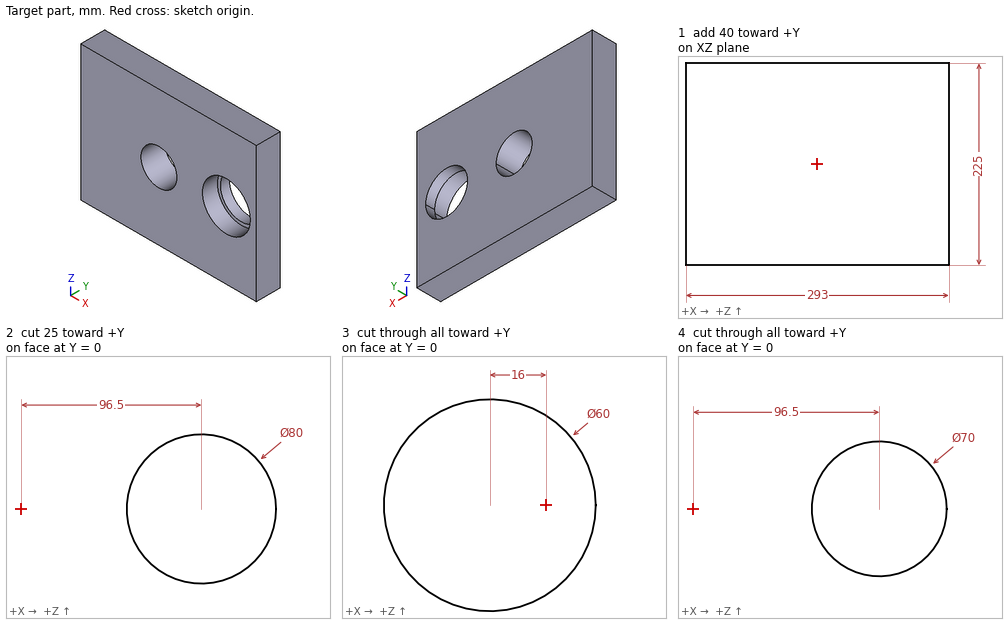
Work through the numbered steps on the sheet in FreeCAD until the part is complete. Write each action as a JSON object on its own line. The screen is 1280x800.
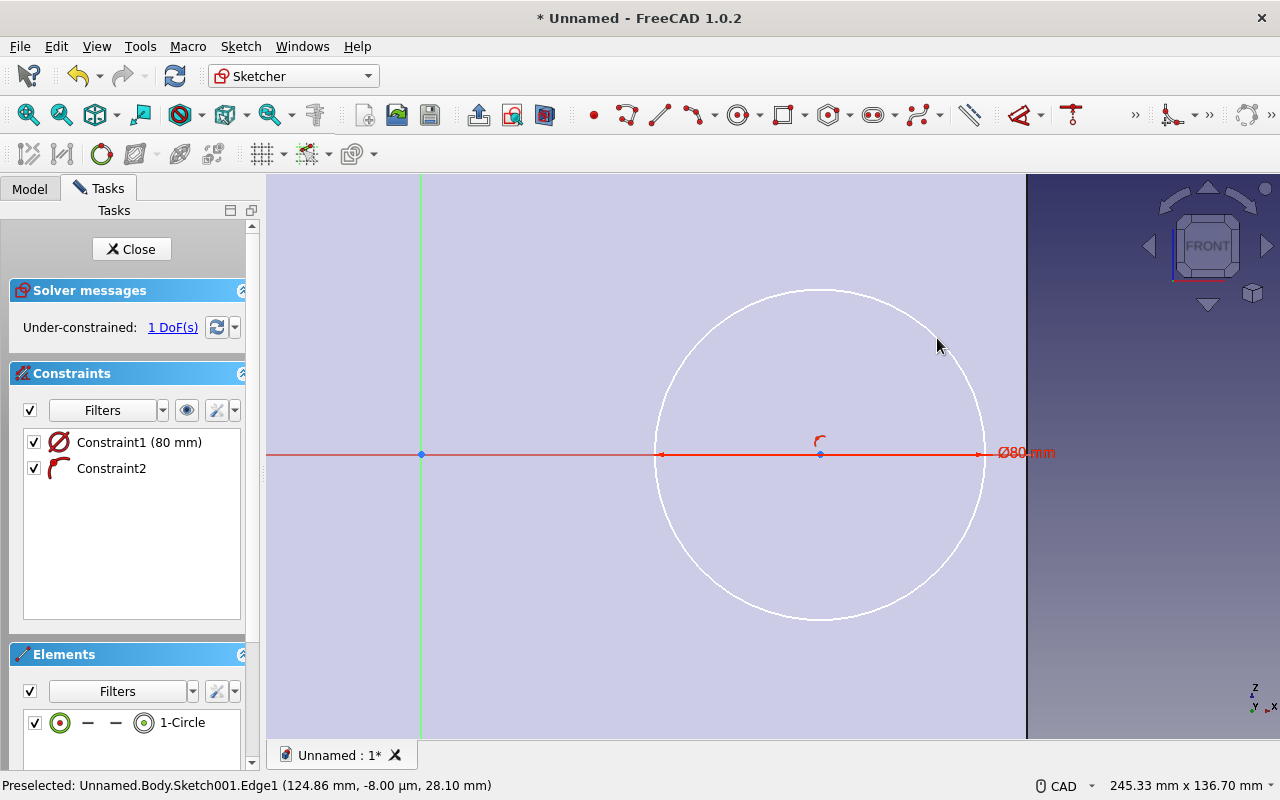
{"action": "left_click", "coordinate": [820, 455]}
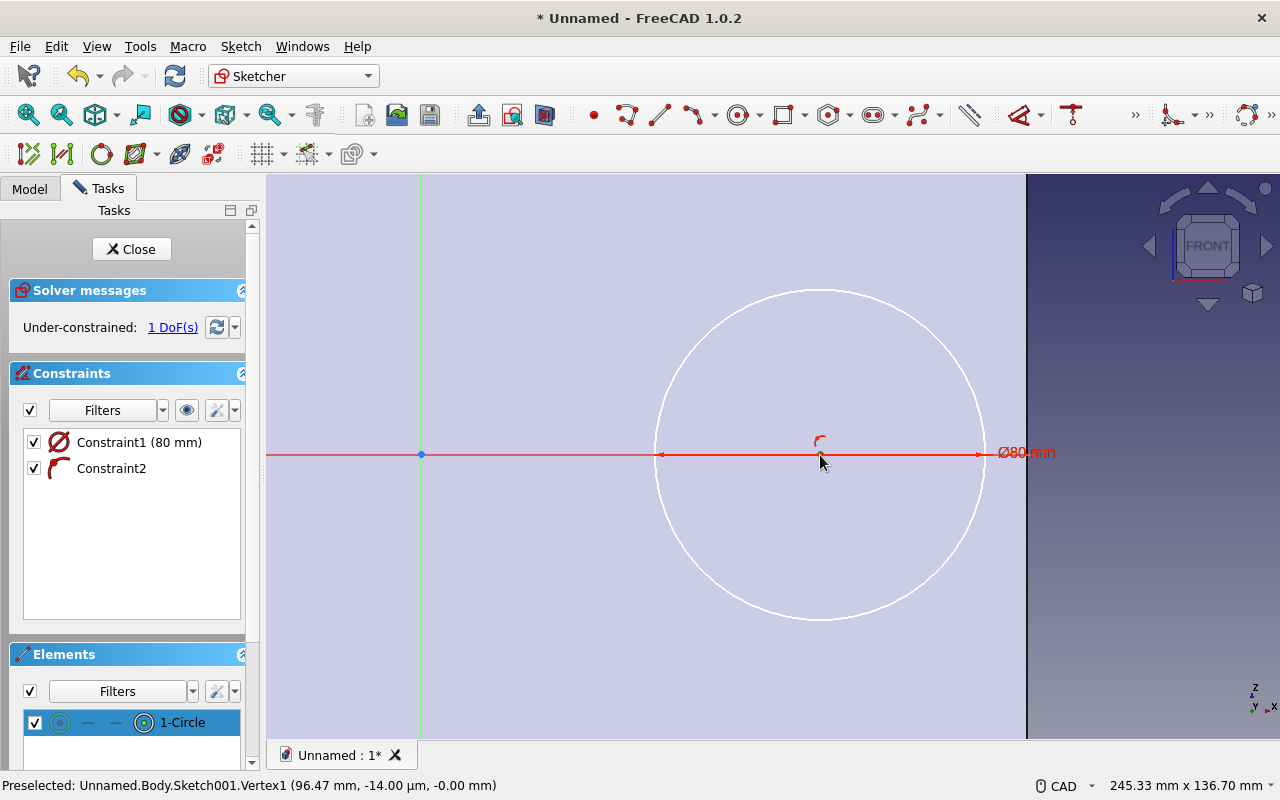
{"action": "left_click", "coordinate": [1040, 116]}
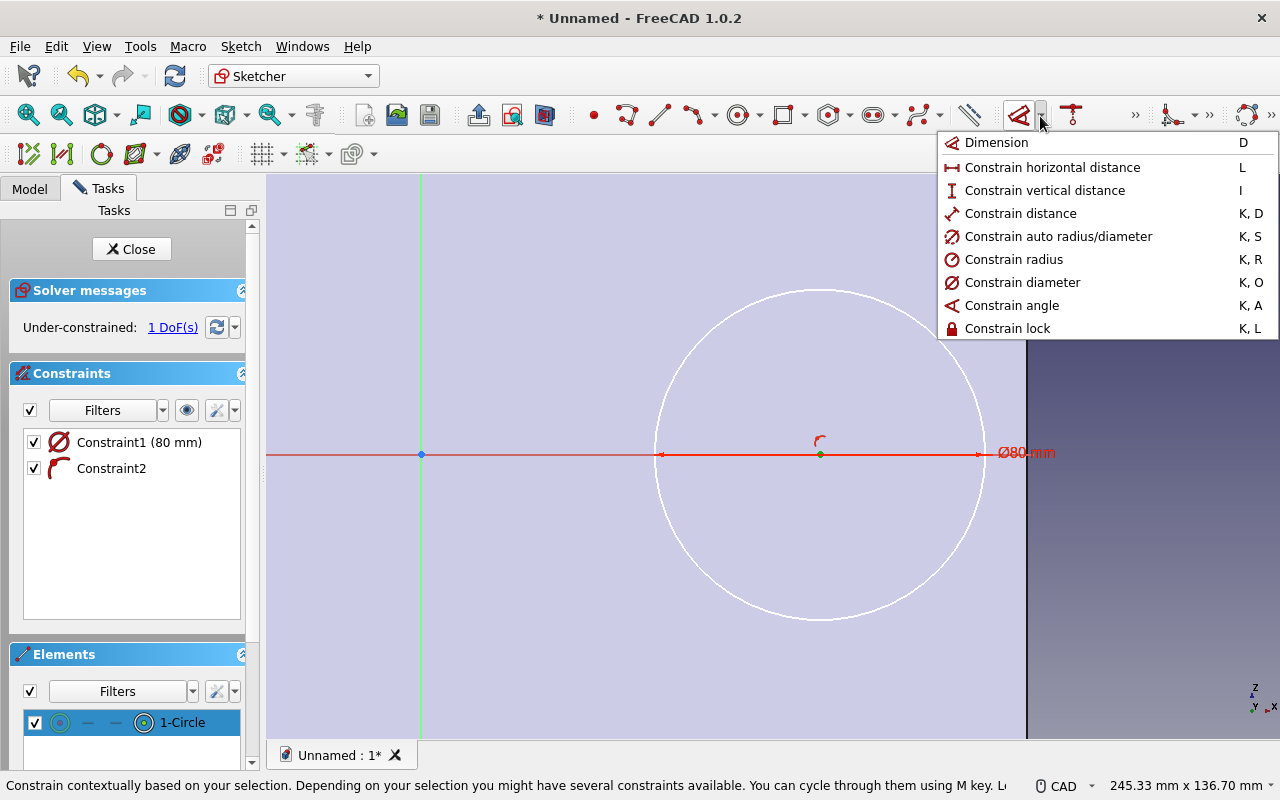
{"action": "left_click", "coordinate": [1108, 168]}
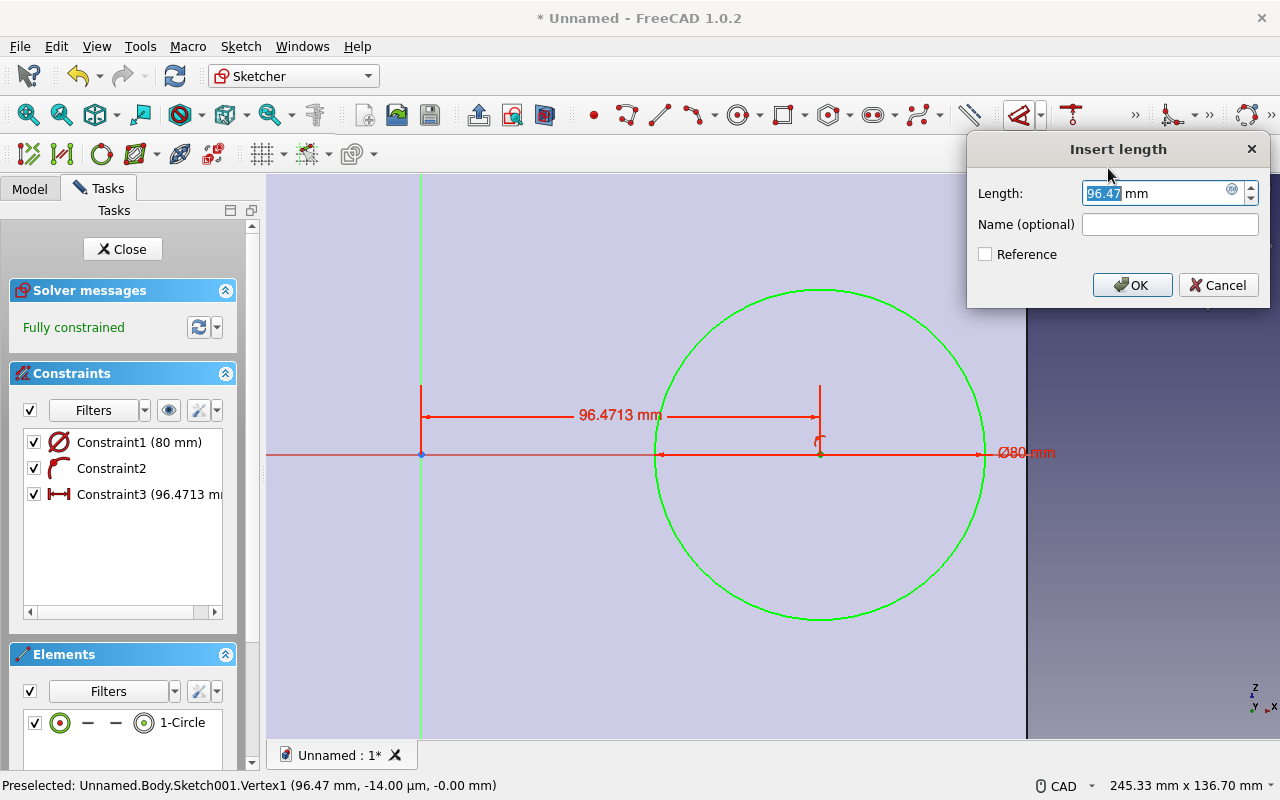
{"action": "type", "text": "96.5"}
{"action": "key", "text": "Return"}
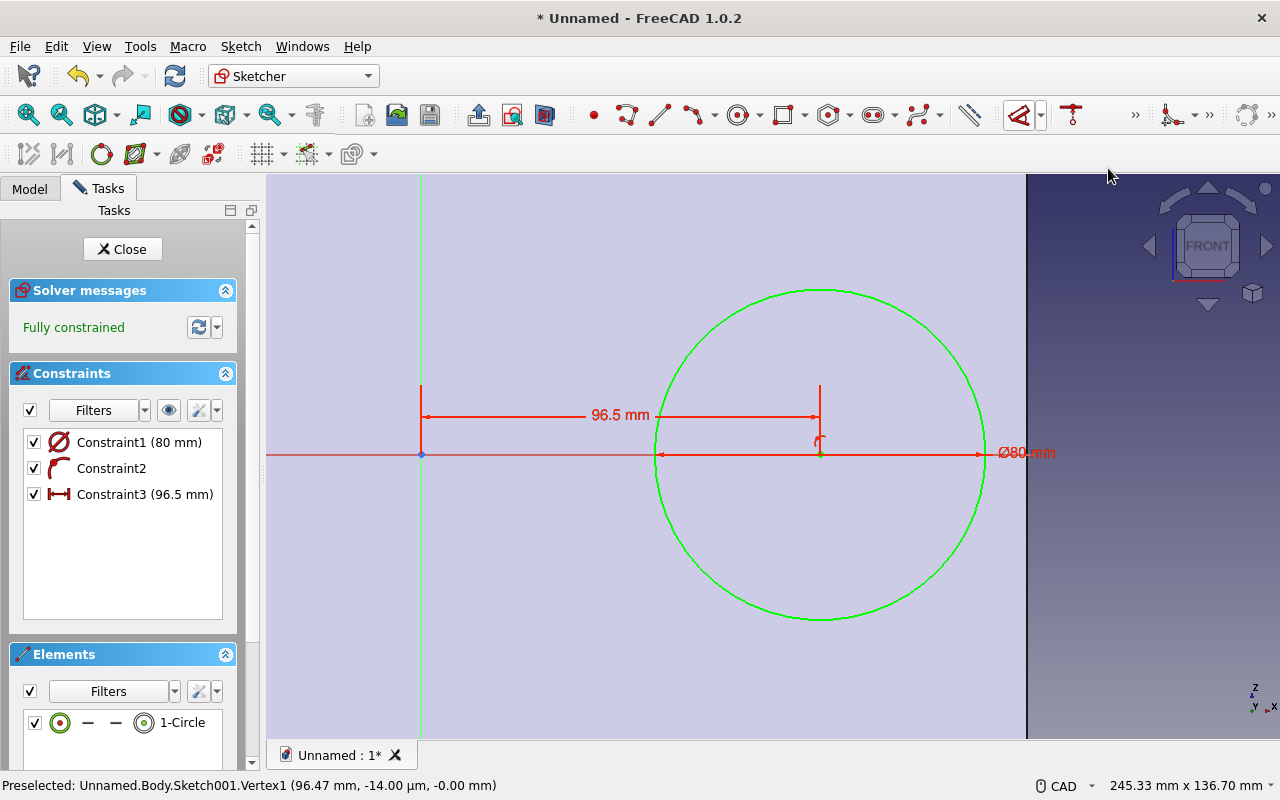
{"action": "left_click", "coordinate": [123, 249]}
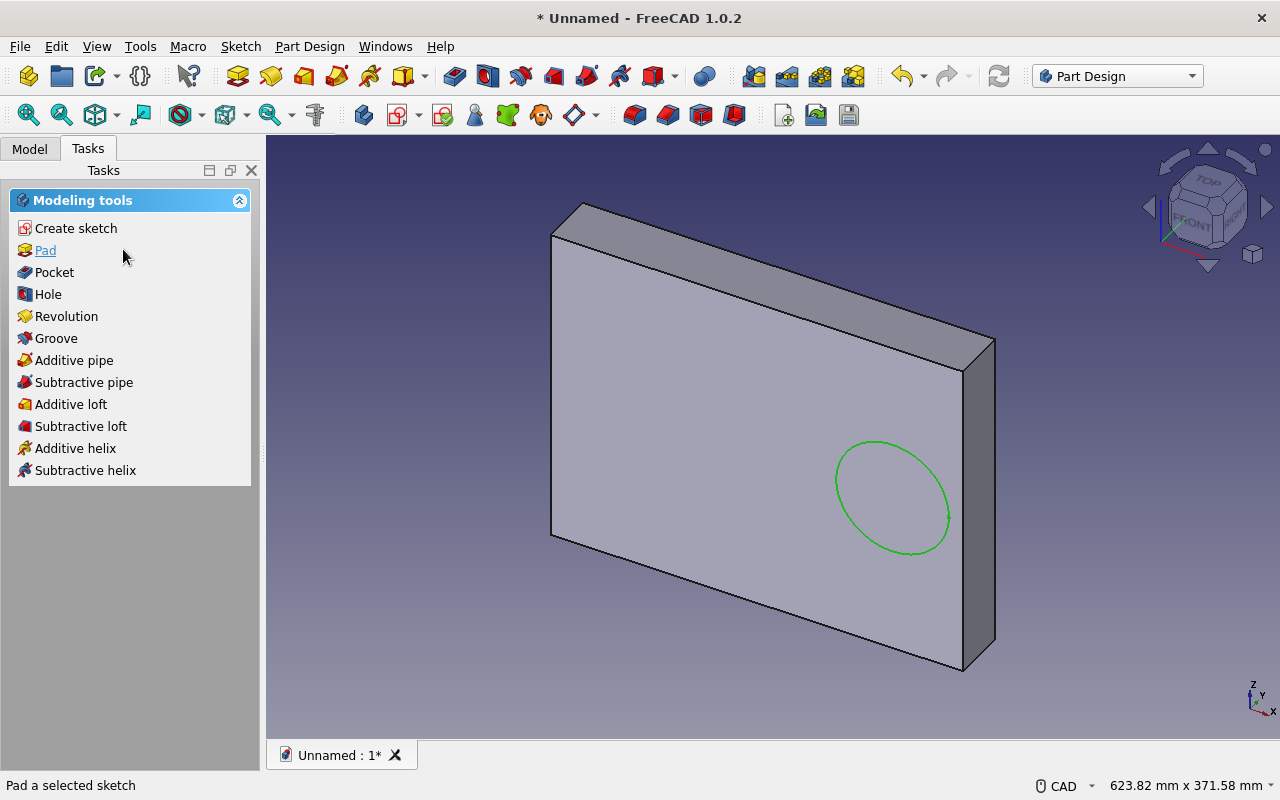
{"action": "left_click", "coordinate": [455, 76]}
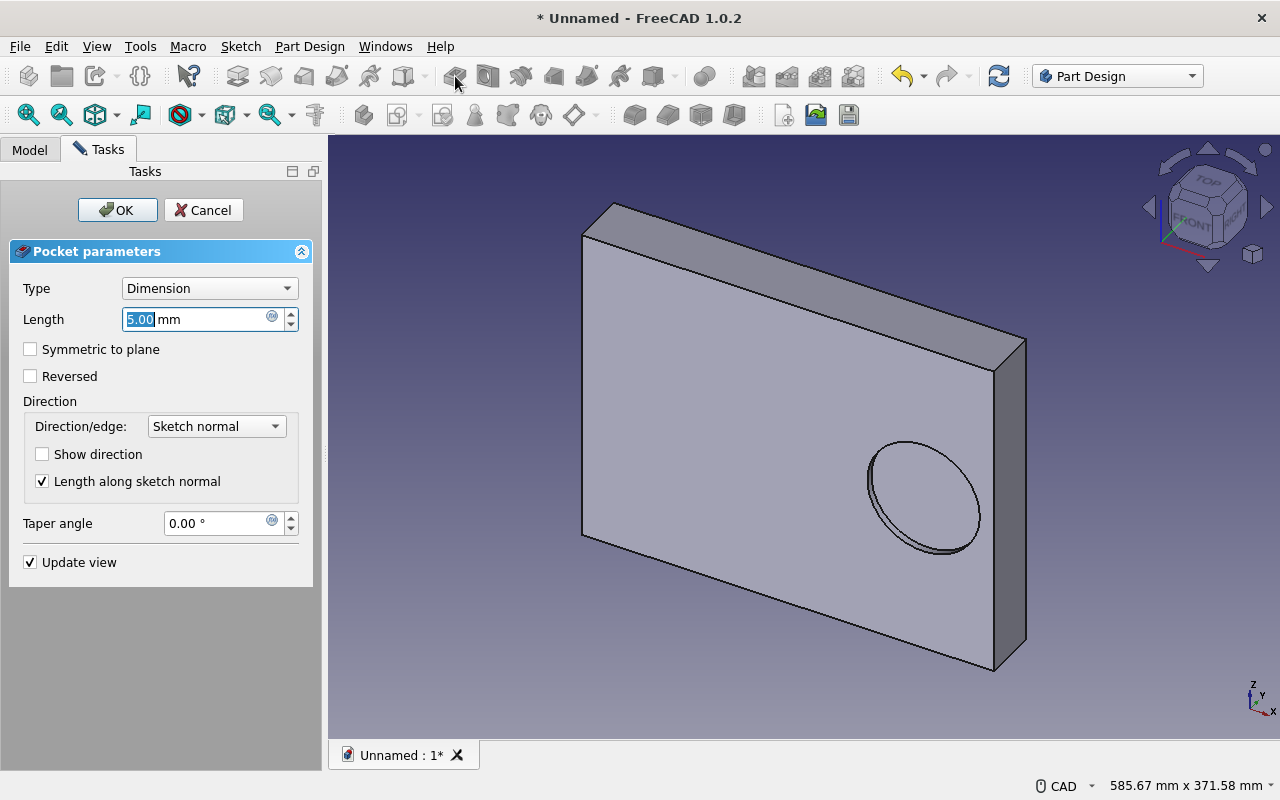
{"action": "type", "text": "25"}
{"action": "key", "text": "Tab"}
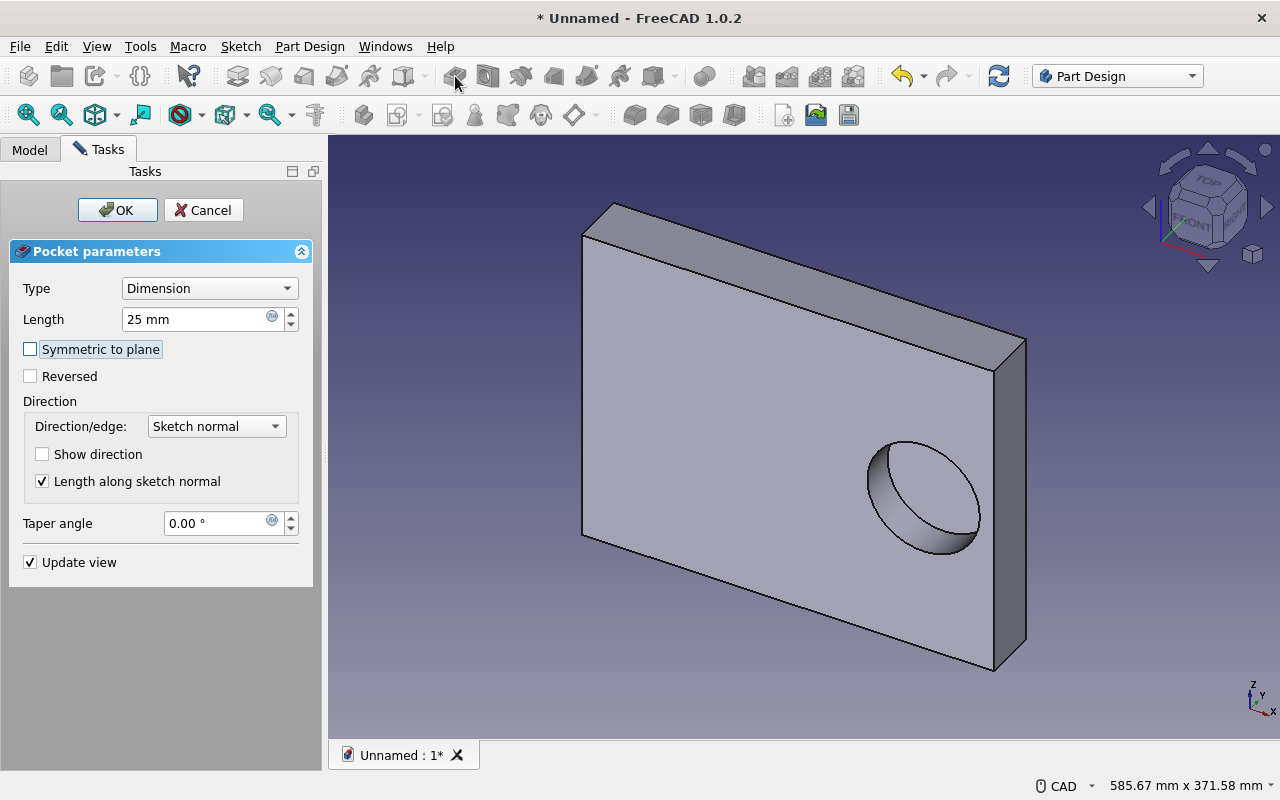
{"action": "left_click", "coordinate": [118, 210]}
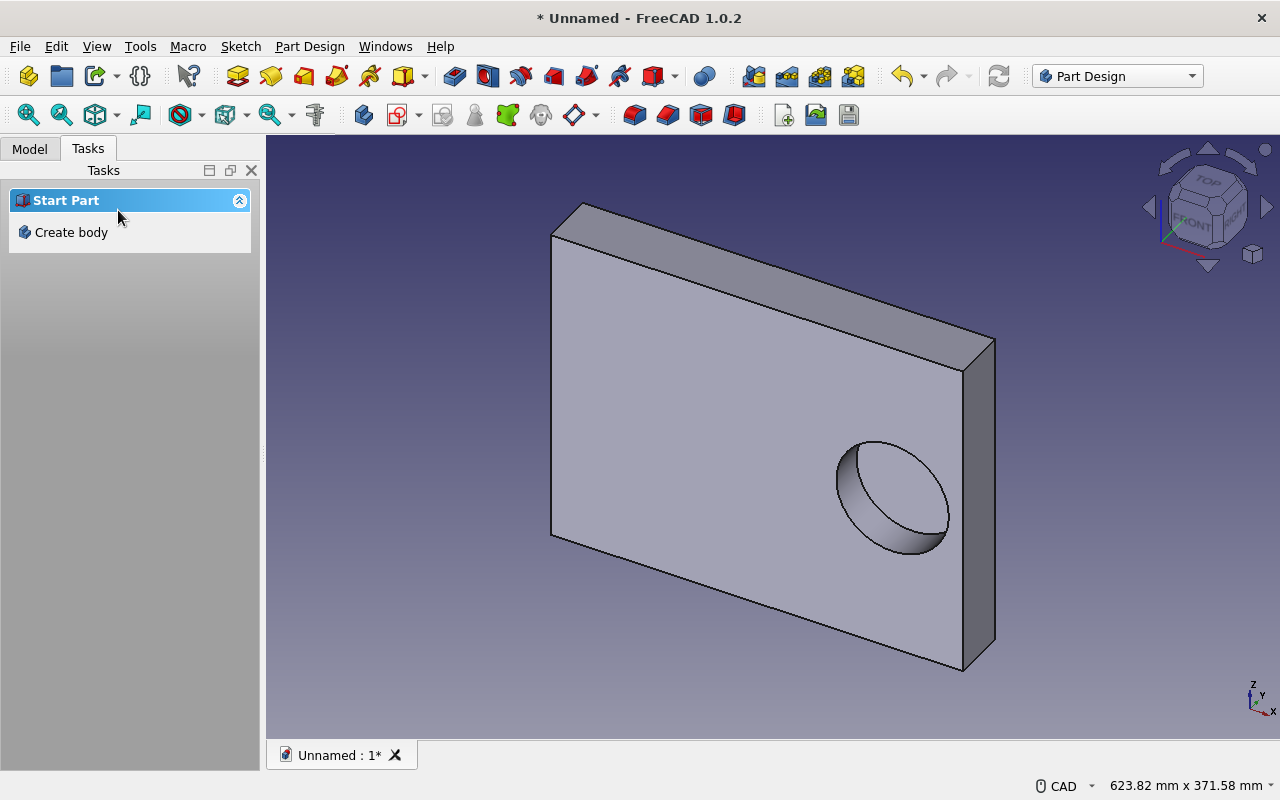
{"action": "left_click", "coordinate": [698, 433]}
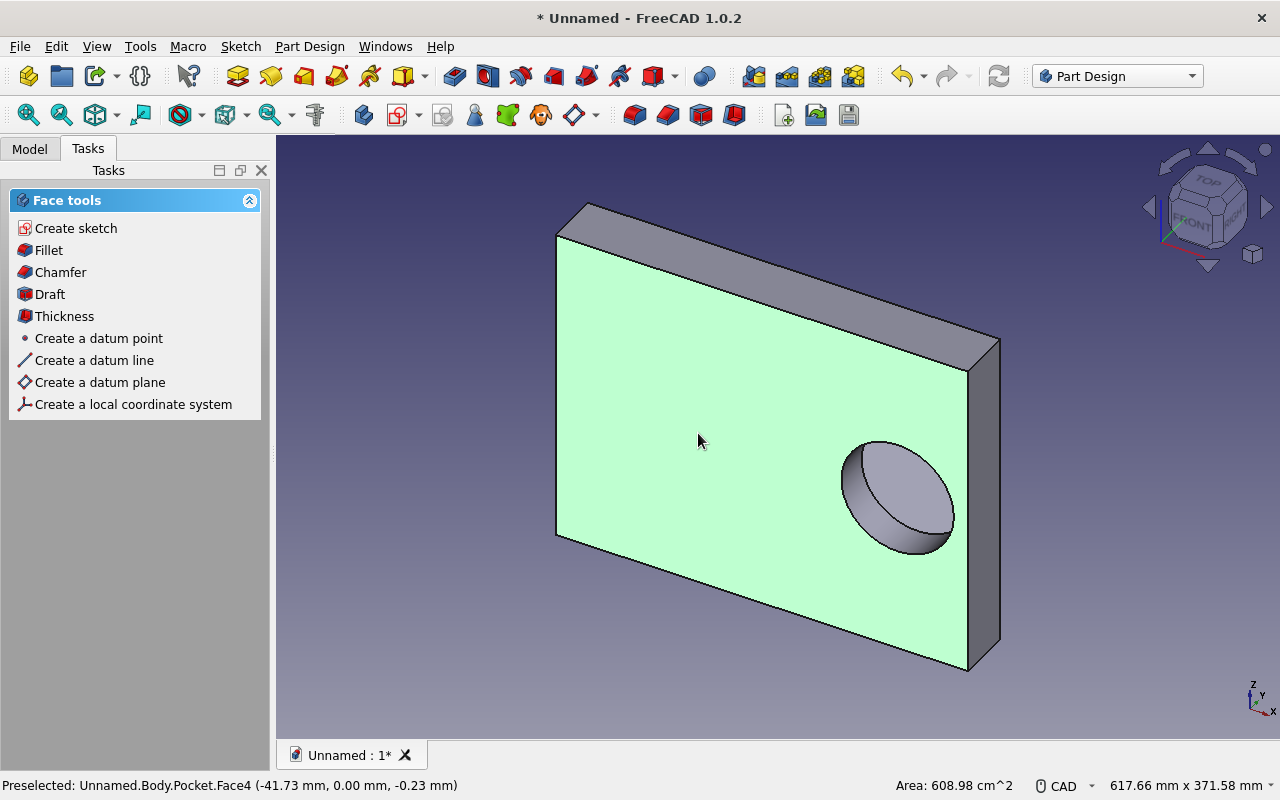
{"action": "left_click", "coordinate": [396, 116]}